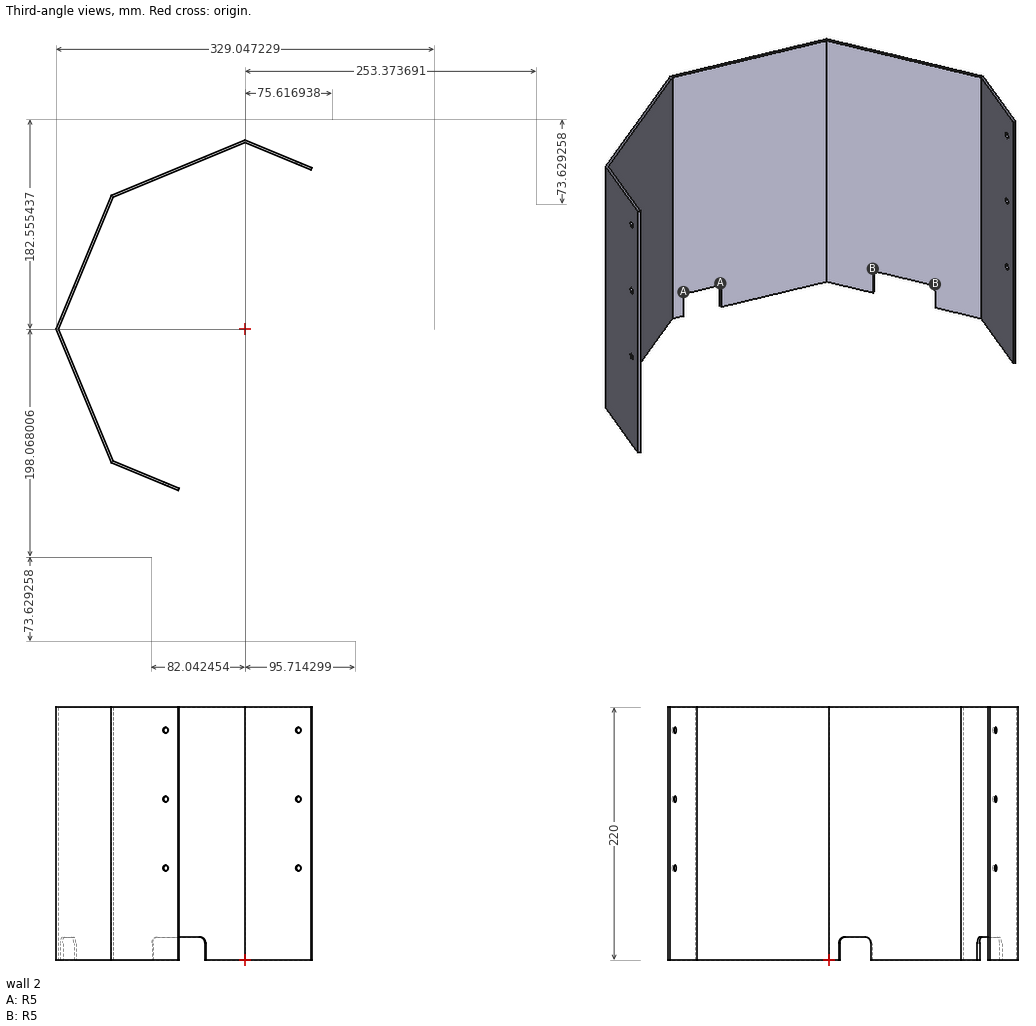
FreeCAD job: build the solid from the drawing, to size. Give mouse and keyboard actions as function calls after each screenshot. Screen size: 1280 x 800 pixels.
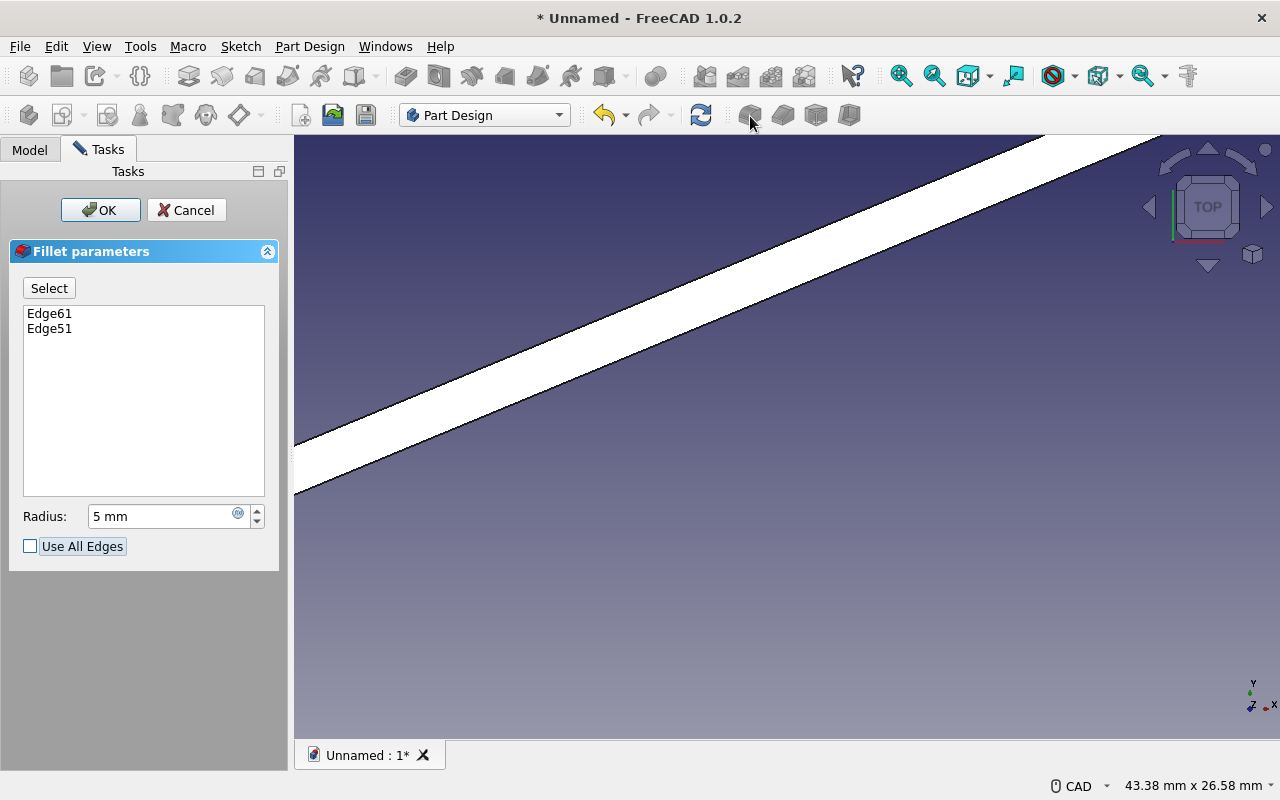
click(101, 210)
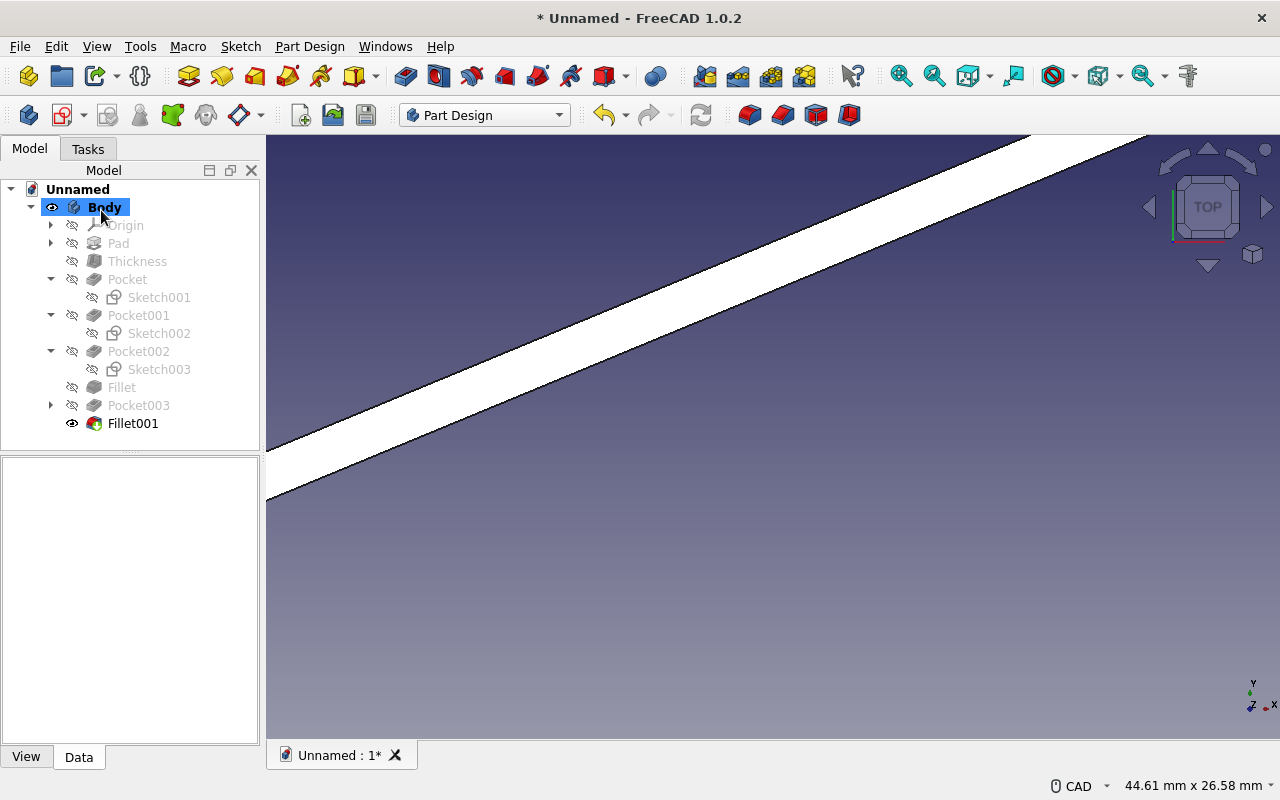
key(0)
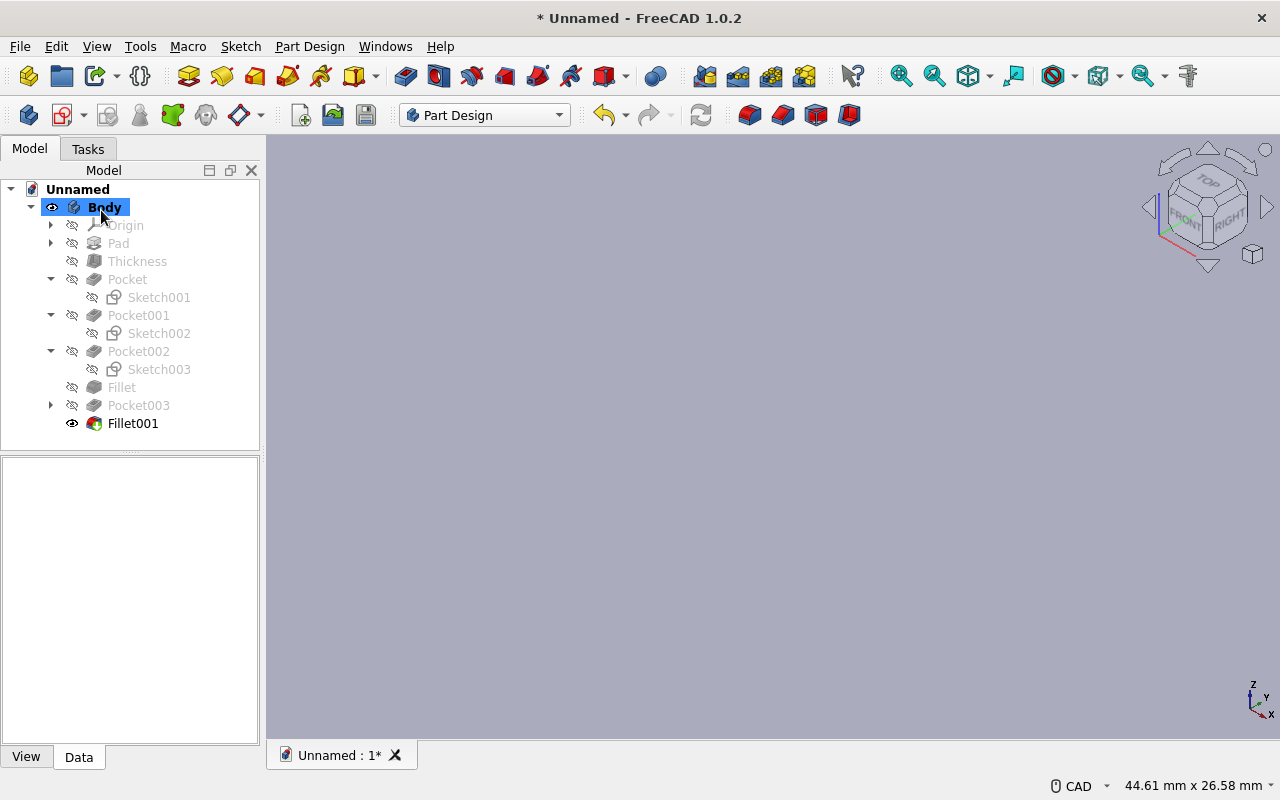
click(902, 76)